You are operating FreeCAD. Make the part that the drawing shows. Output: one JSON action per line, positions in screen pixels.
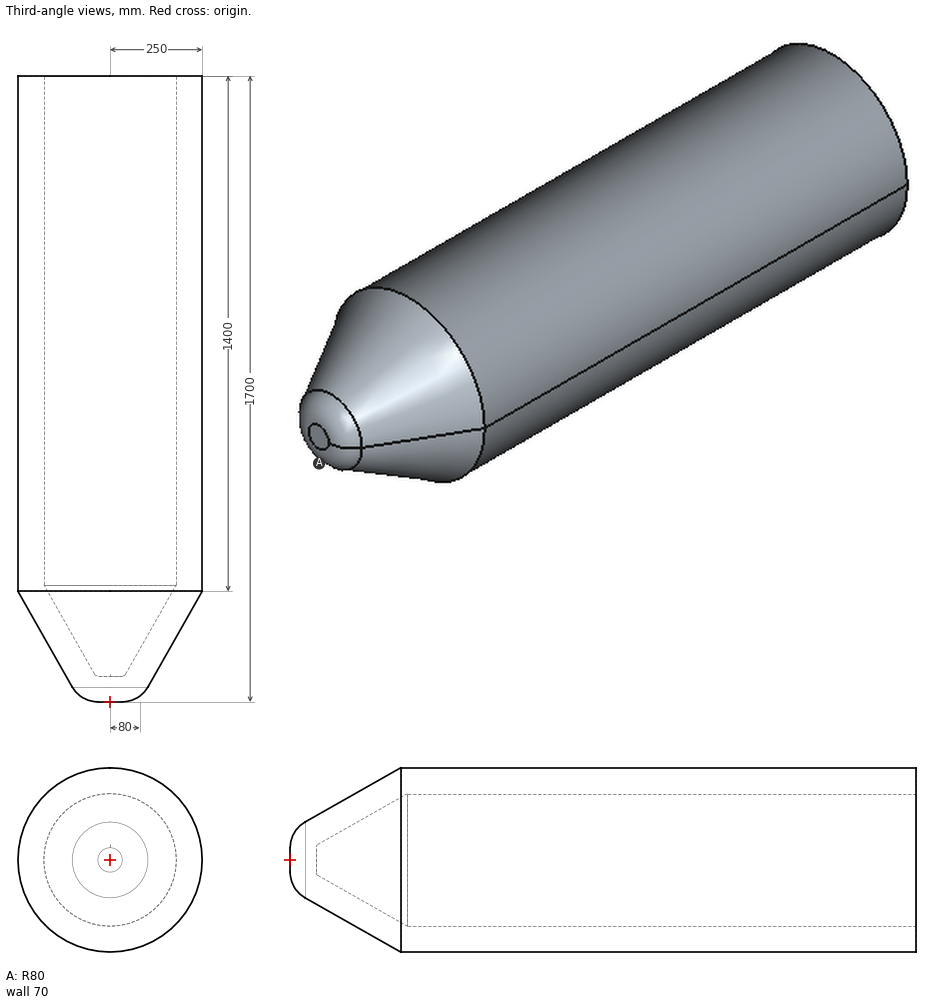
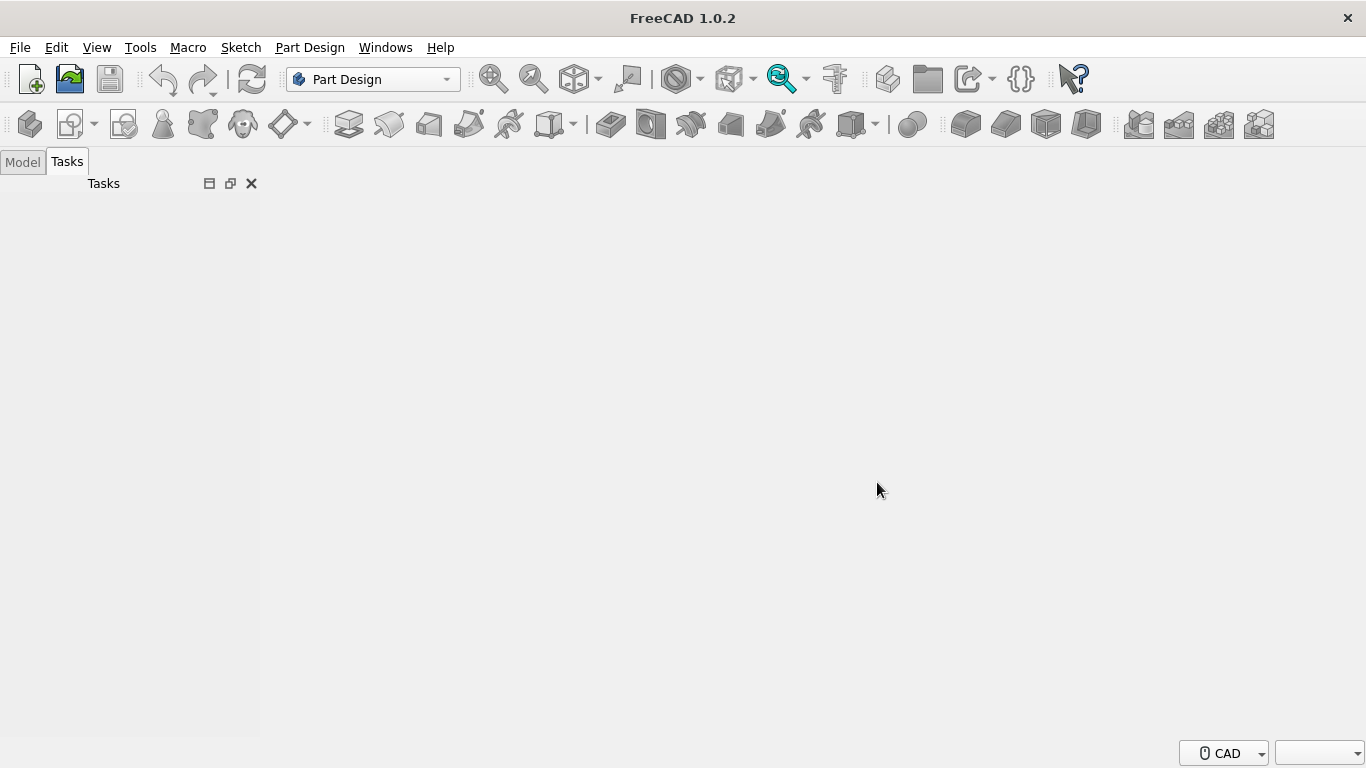
{"action": "left_click", "coordinate": [30, 80]}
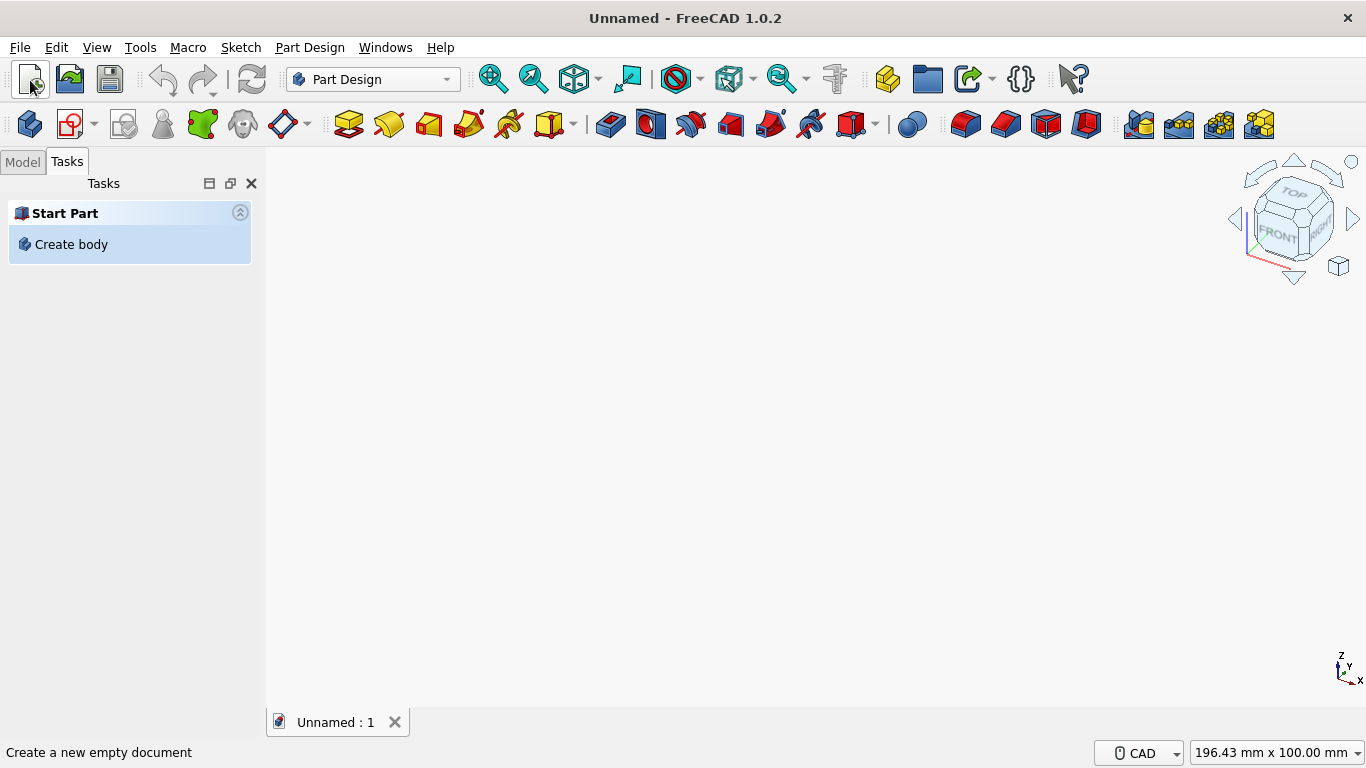
{"action": "left_click", "coordinate": [70, 124]}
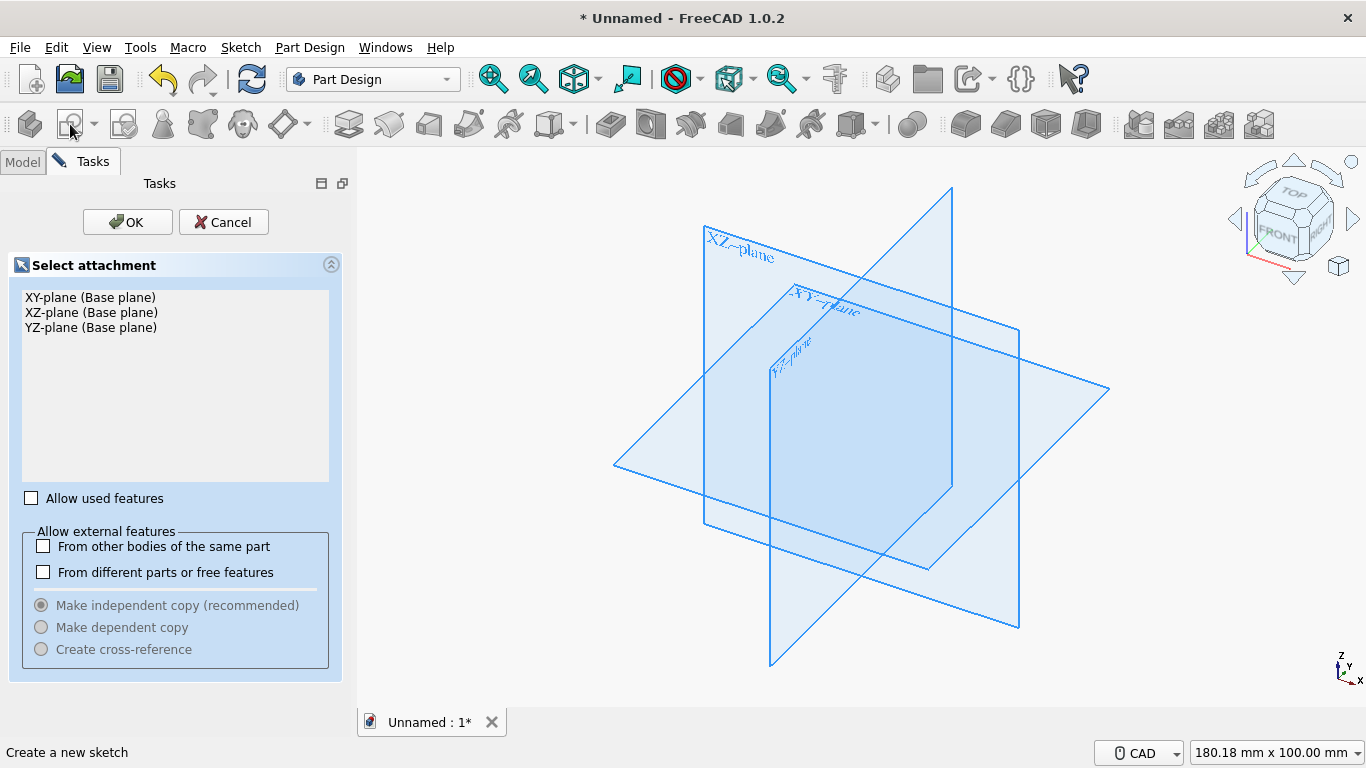
{"action": "left_click", "coordinate": [82, 298]}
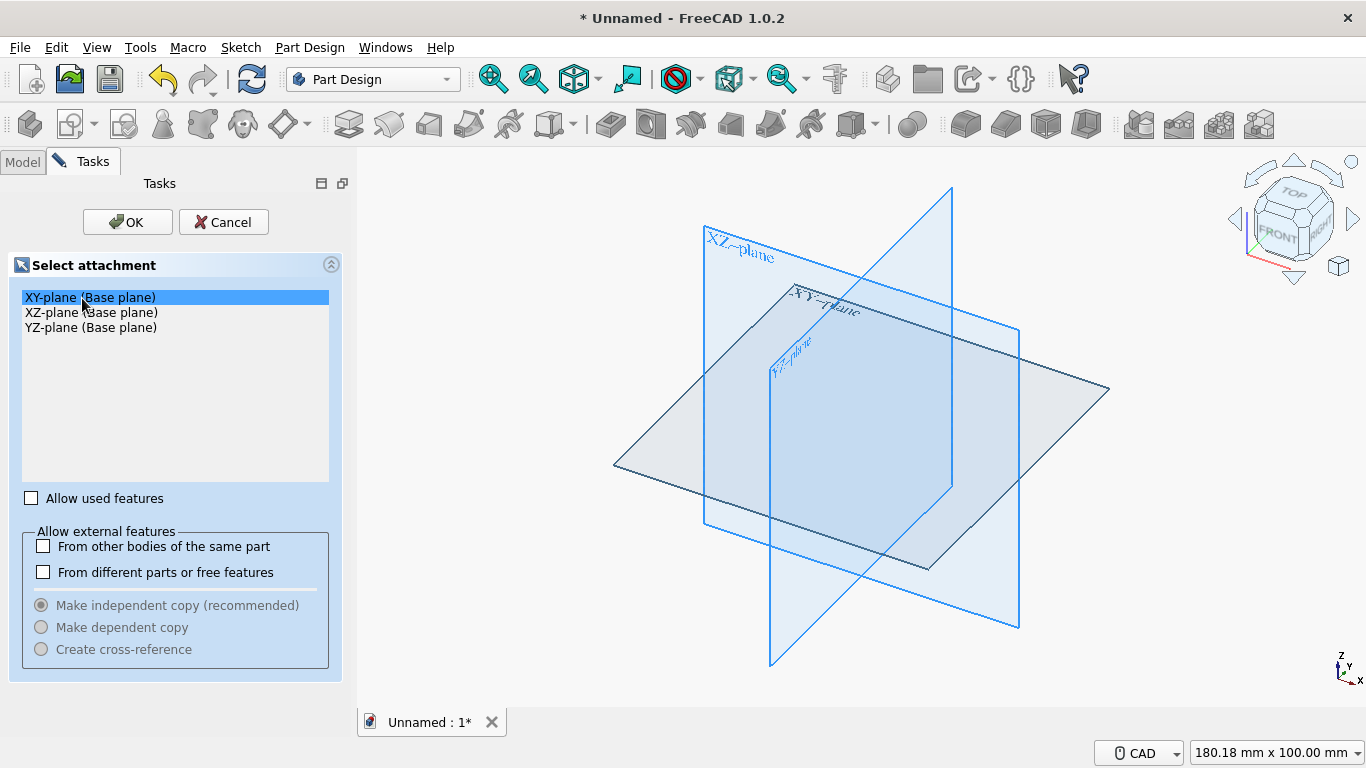
{"action": "left_click", "coordinate": [128, 222]}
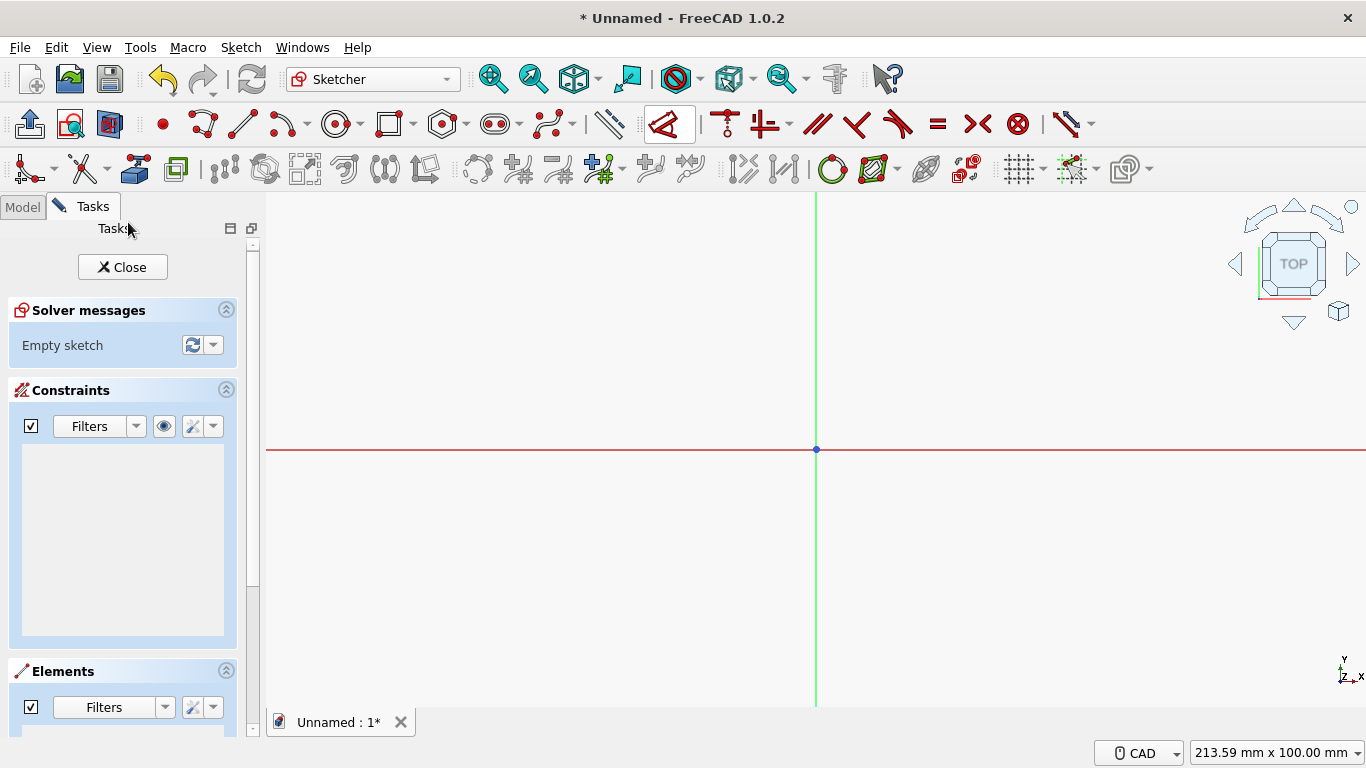
{"action": "scroll", "coordinate": [717, 636], "scroll_direction": "down", "scroll_amount": 16}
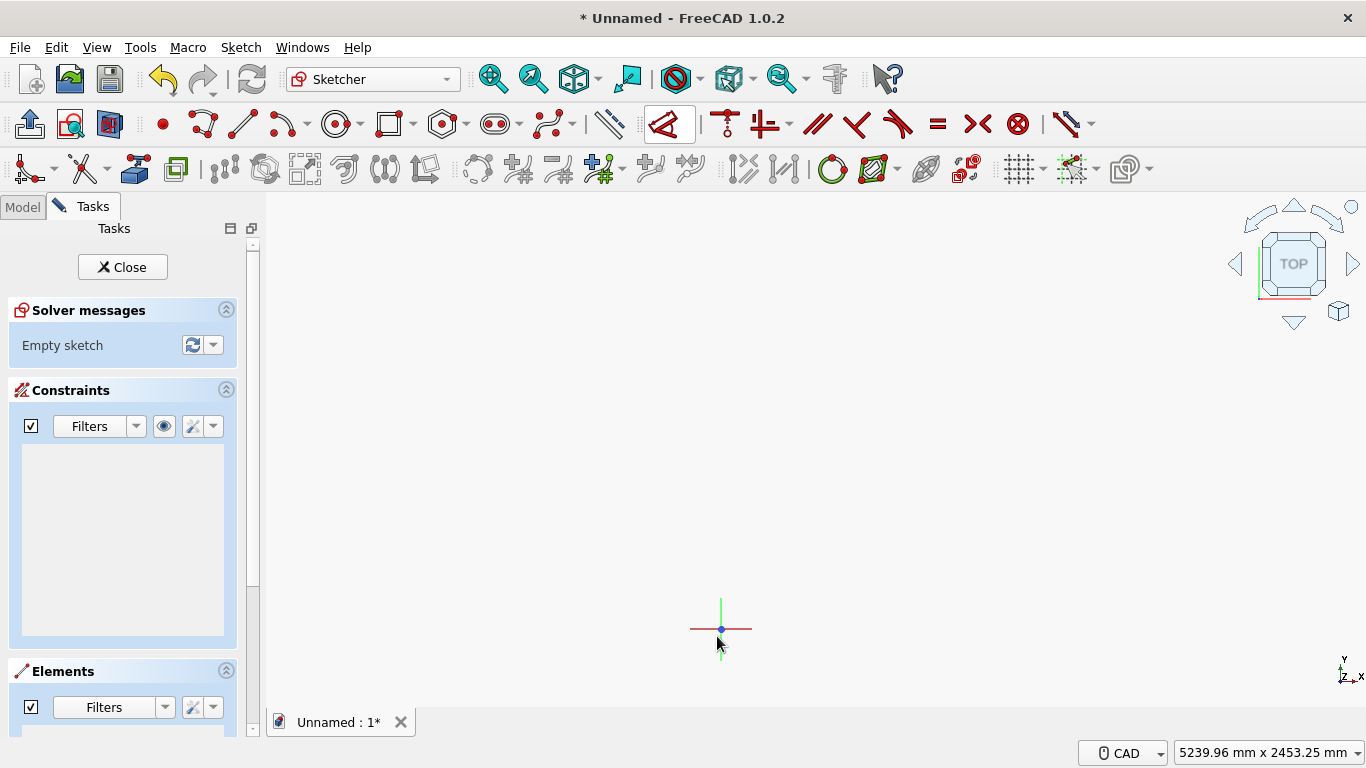
{"action": "left_click", "coordinate": [204, 124]}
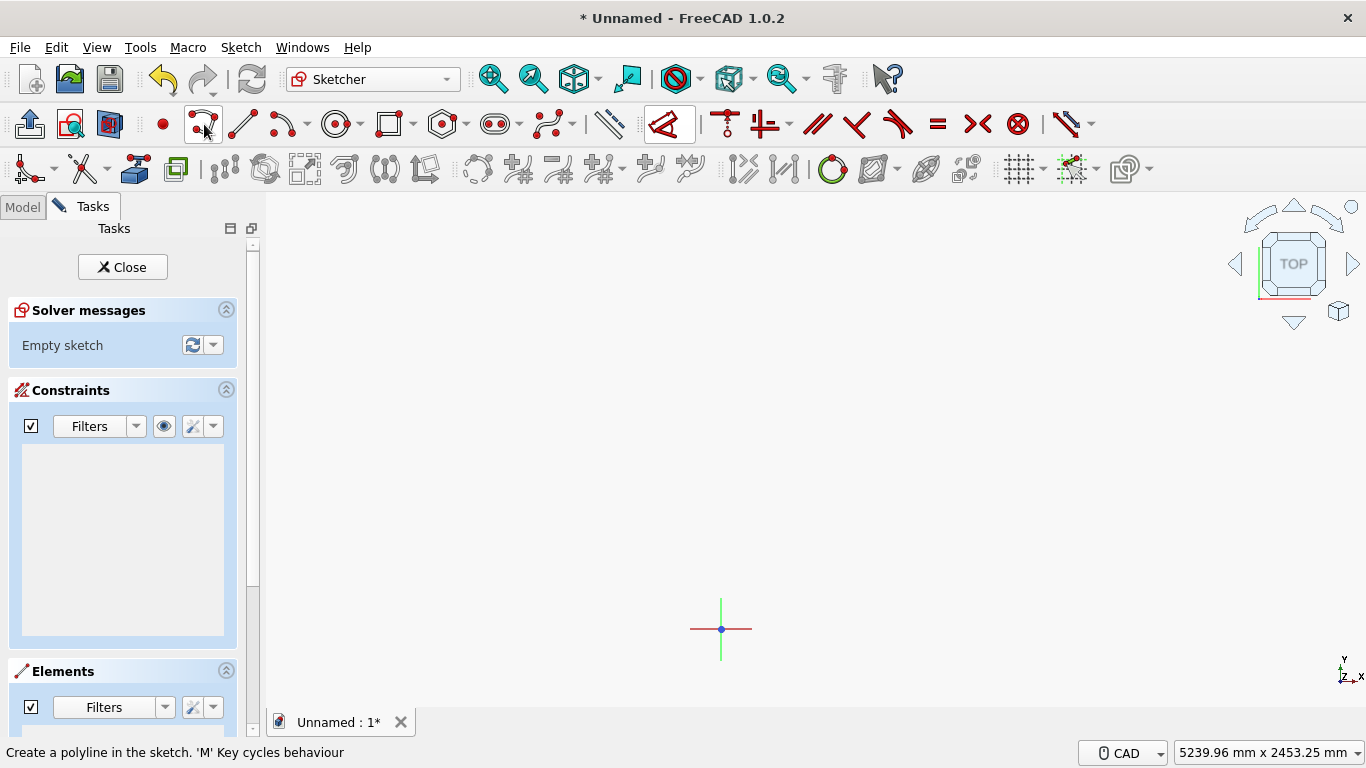
{"action": "left_click", "coordinate": [721, 629]}
{"action": "left_click", "coordinate": [738, 620]}
{"action": "left_click", "coordinate": [774, 566]}
{"action": "left_click", "coordinate": [774, 272]}
{"action": "left_click", "coordinate": [730, 272]}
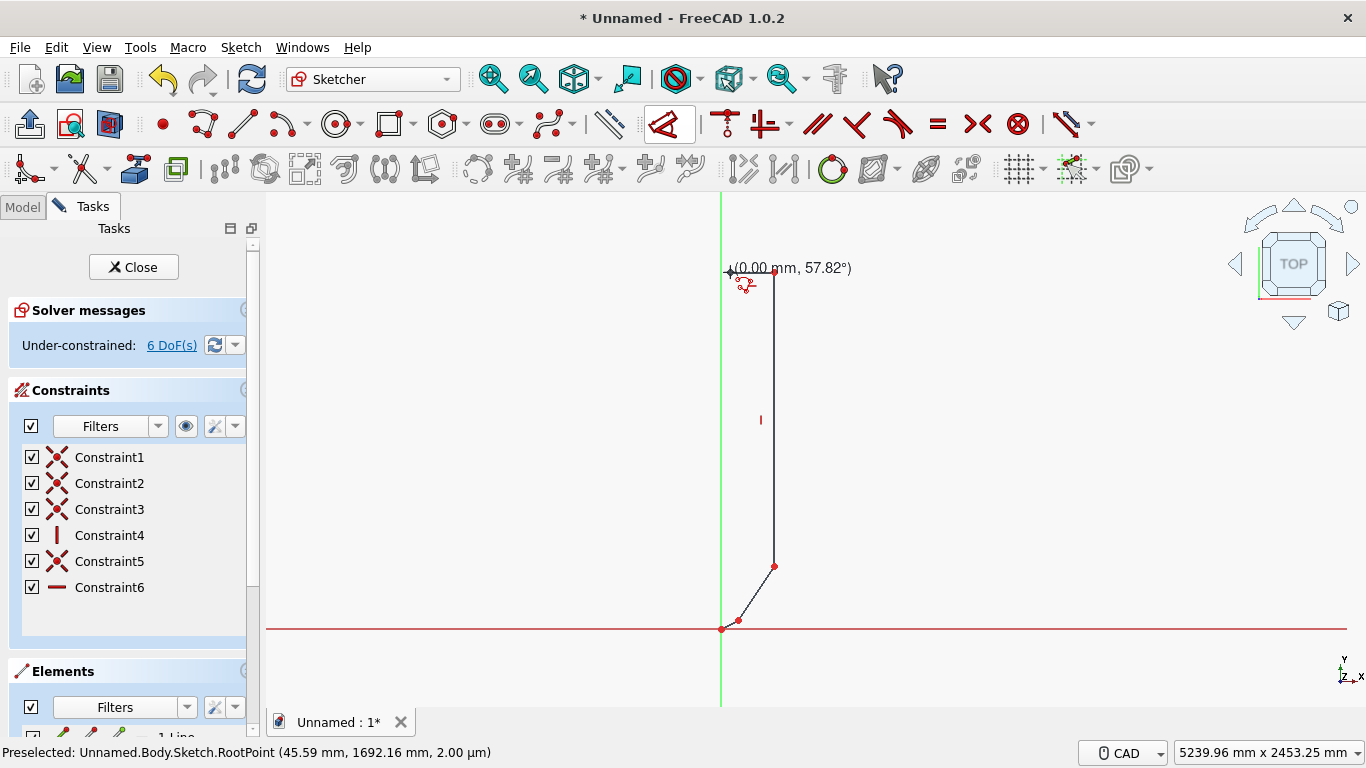
{"action": "scroll", "coordinate": [721, 629], "scroll_direction": "up", "scroll_amount": 4}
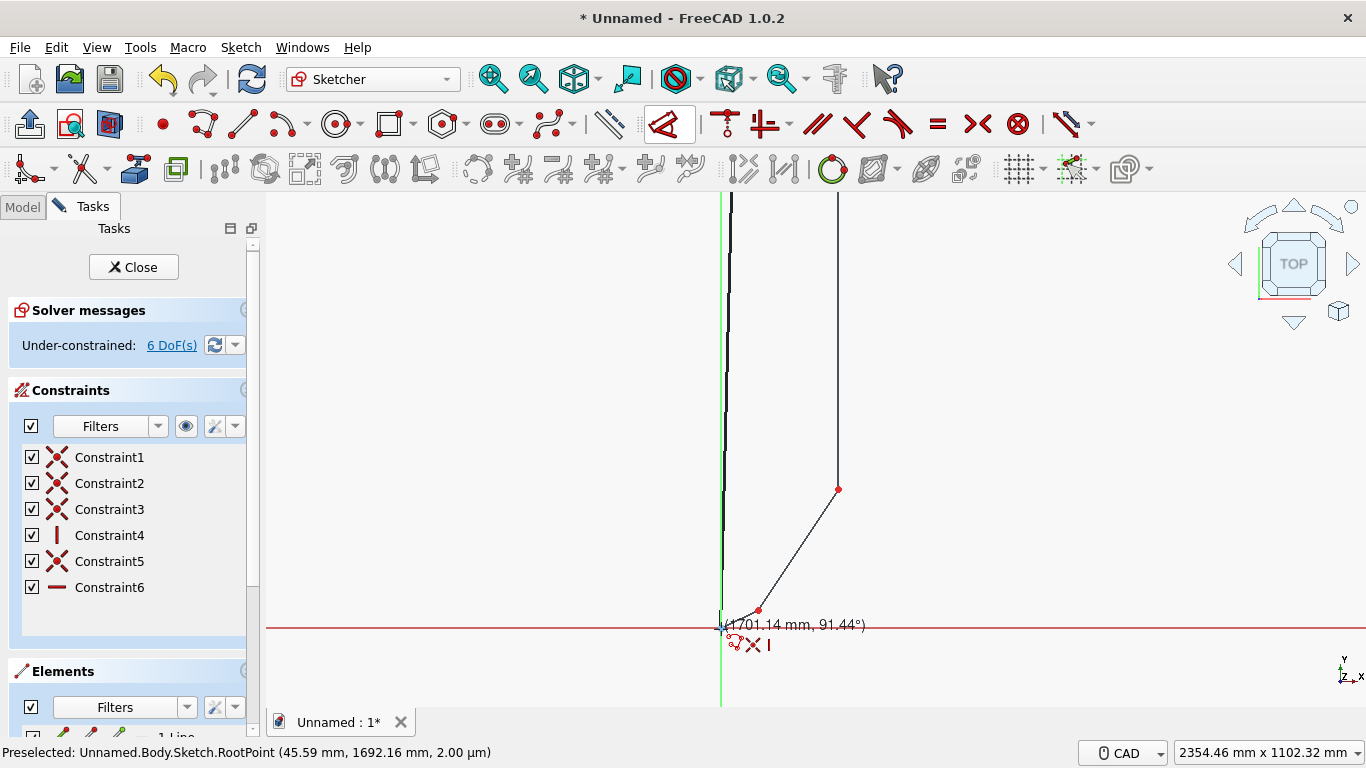
{"action": "left_click", "coordinate": [721, 628]}
{"action": "key", "text": "Escape"}
{"action": "key", "text": "Escape"}